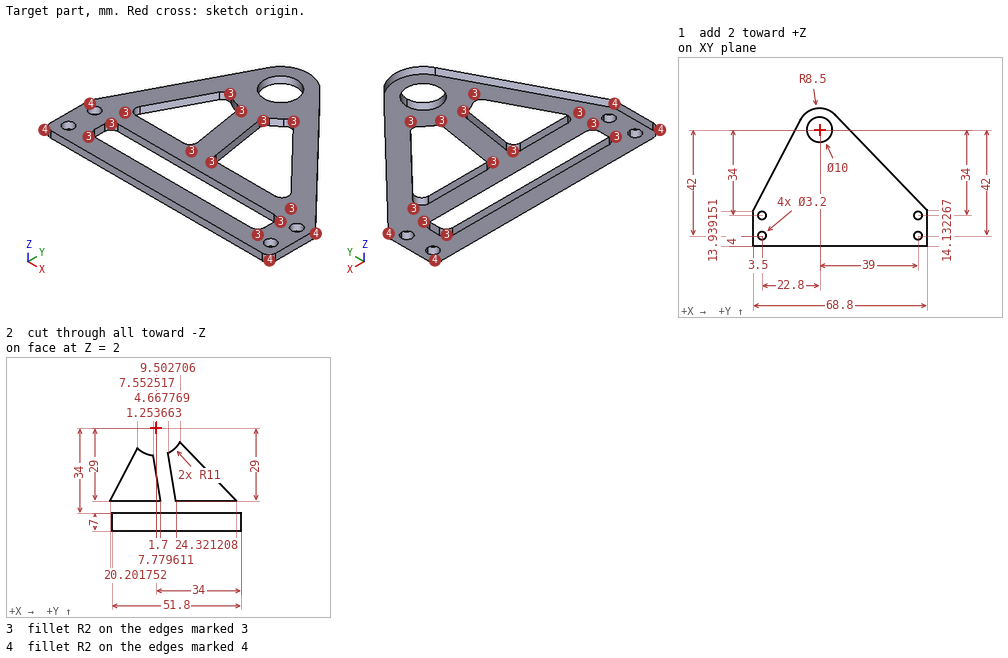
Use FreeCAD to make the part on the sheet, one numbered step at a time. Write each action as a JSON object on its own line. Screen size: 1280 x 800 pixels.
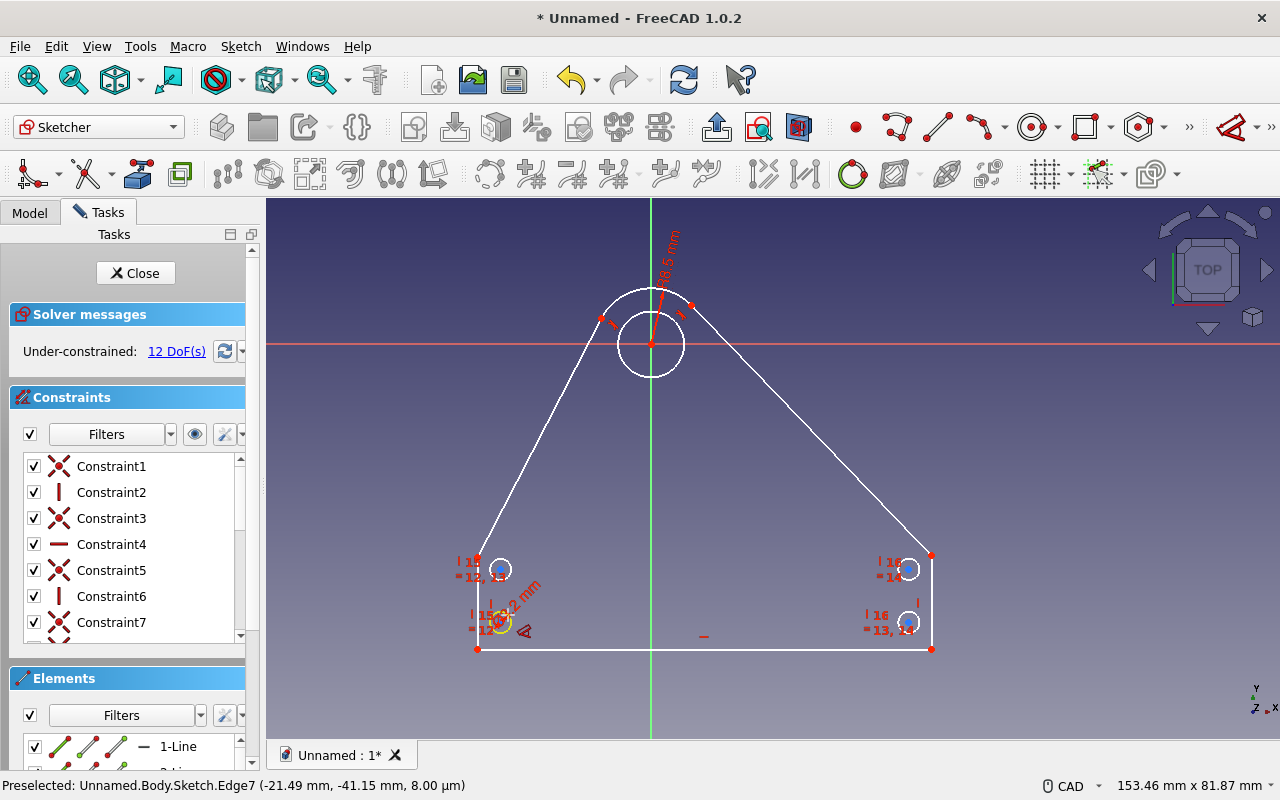
{"action": "left_click", "coordinate": [674, 321]}
{"action": "left_click", "coordinate": [698, 390]}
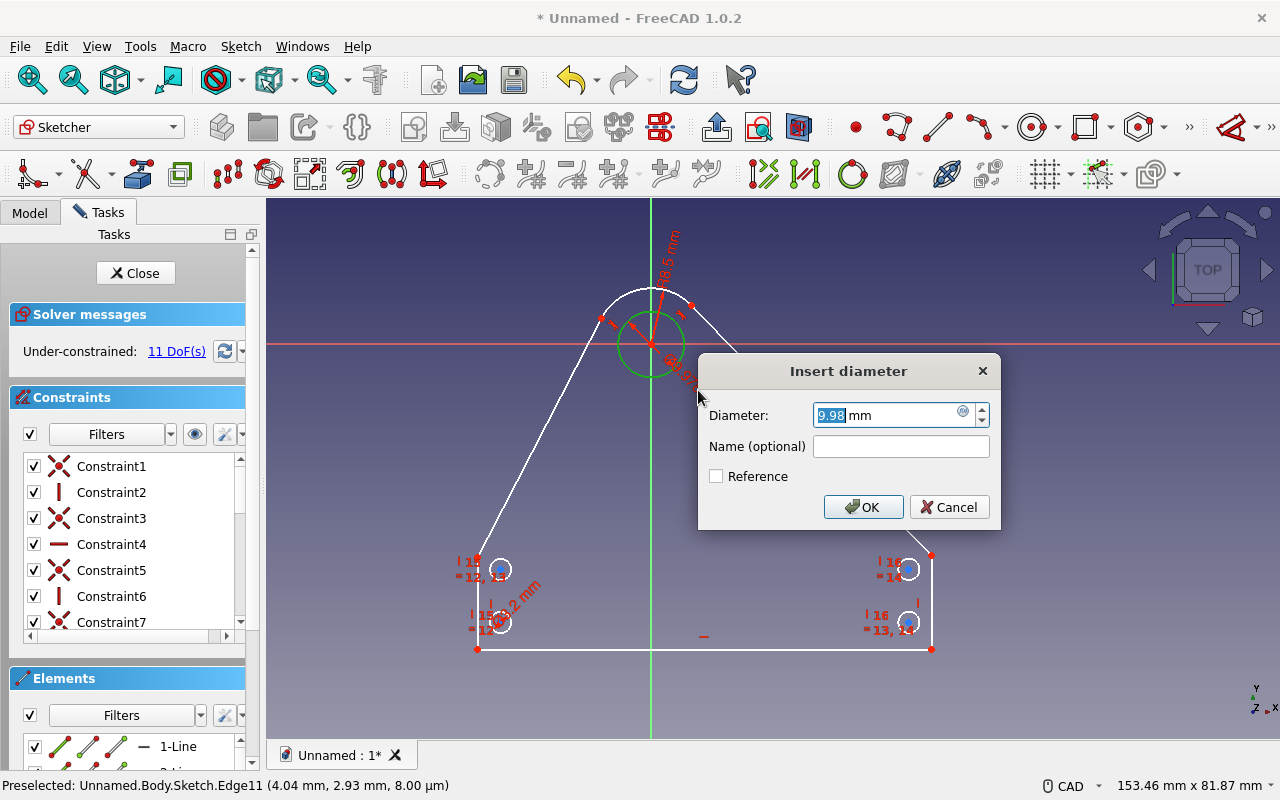
{"action": "type", "text": "10"}
{"action": "key", "text": "Return"}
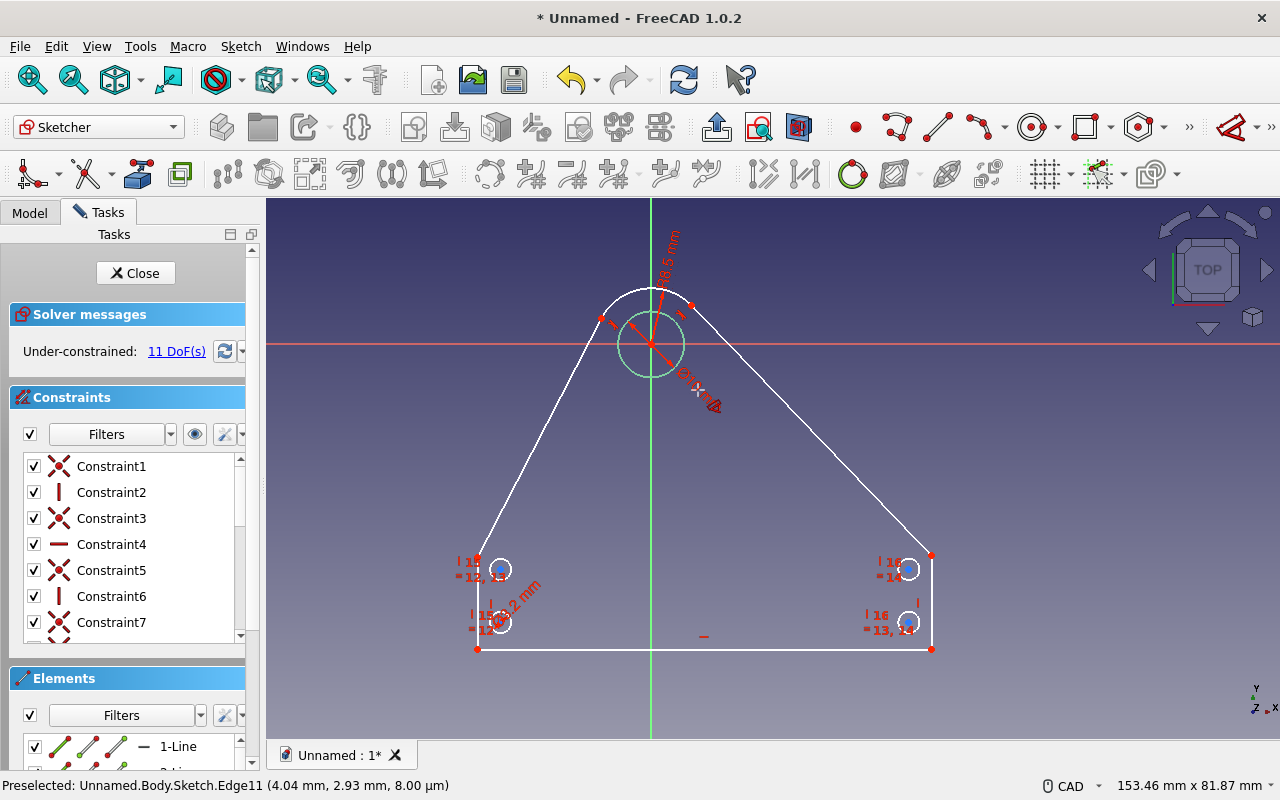
{"action": "left_click", "coordinate": [501, 623]}
{"action": "left_click", "coordinate": [467, 484]}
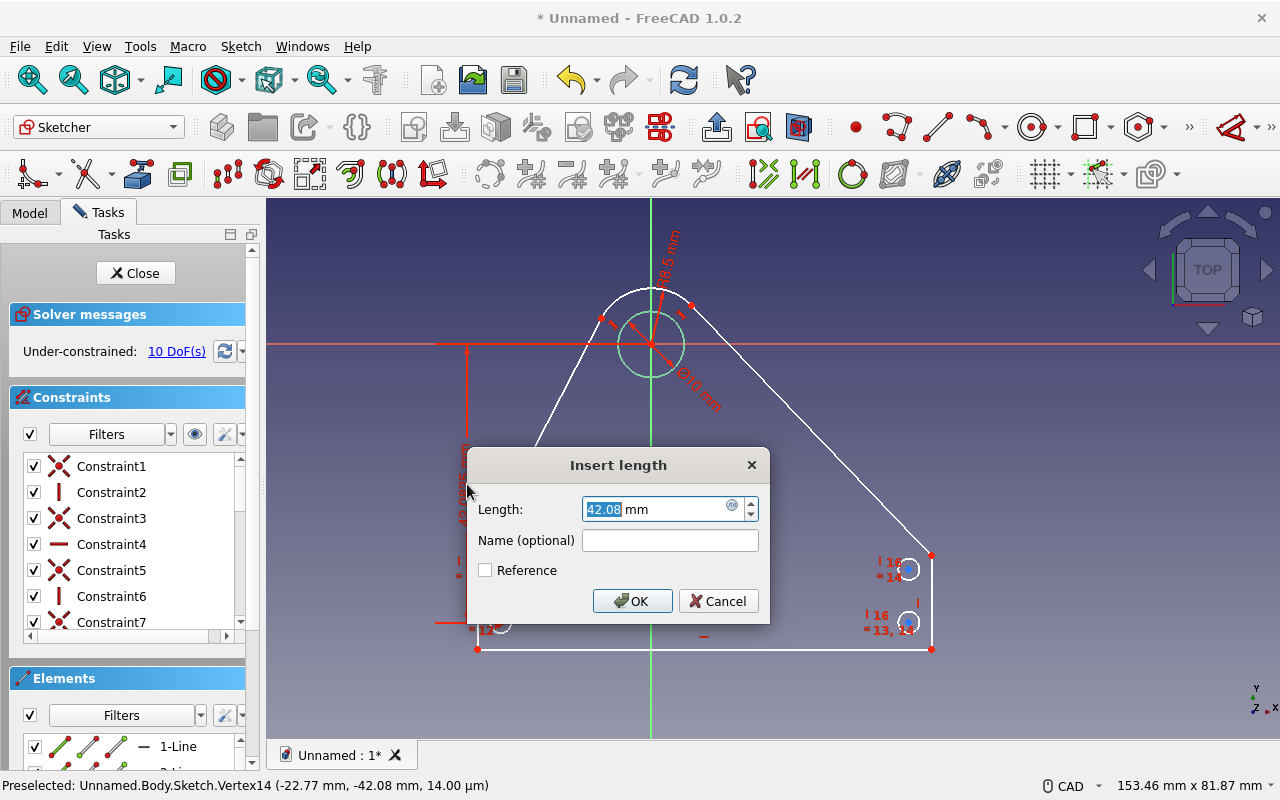
{"action": "type", "text": "42"}
{"action": "key", "text": "Return"}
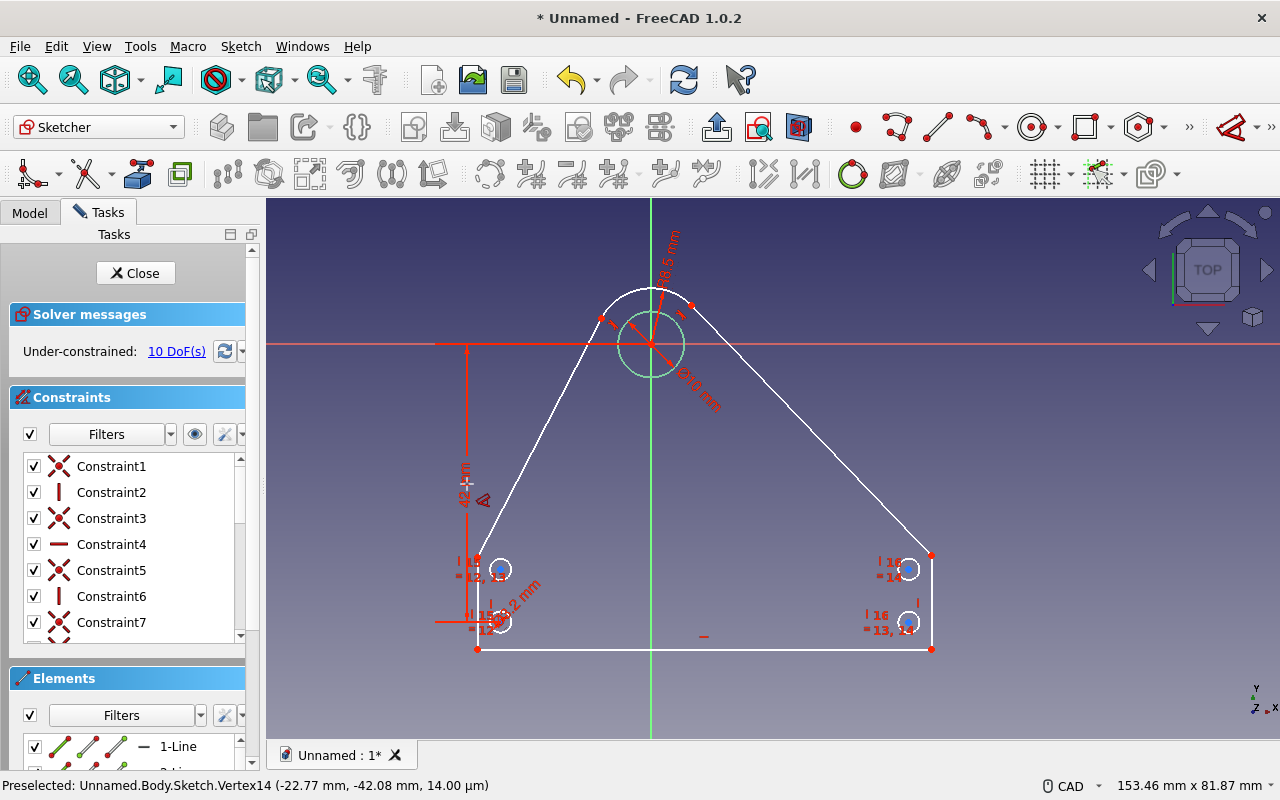
{"action": "left_click", "coordinate": [501, 570]}
{"action": "left_click", "coordinate": [467, 457]}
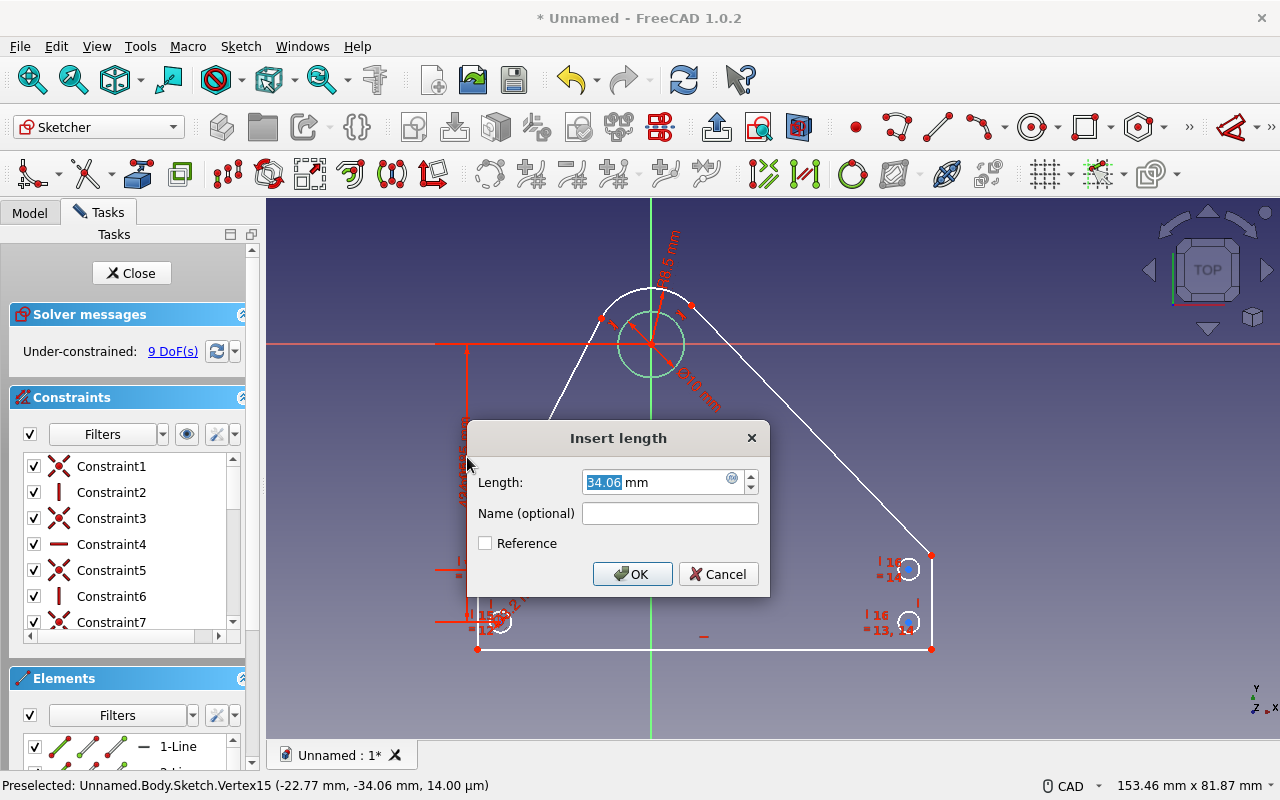
{"action": "type", "text": "34"}
{"action": "key", "text": "Return"}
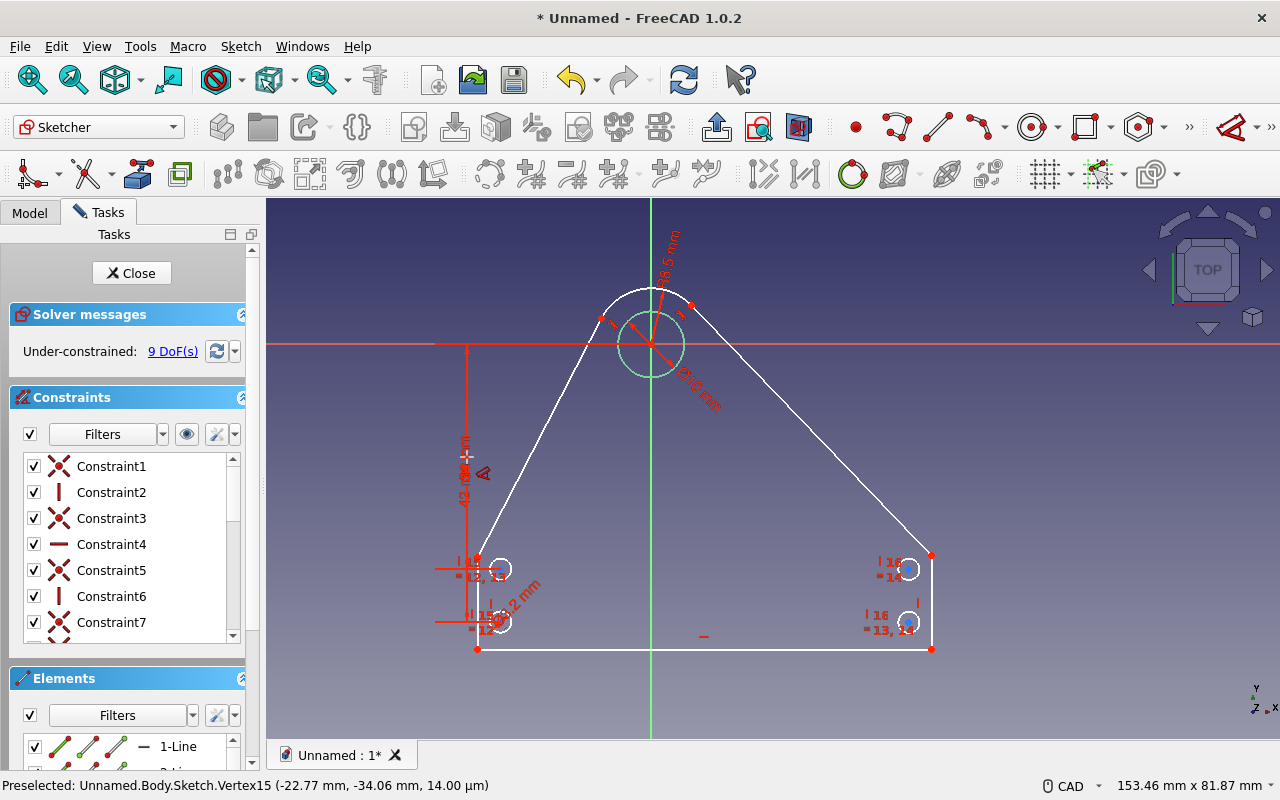
{"action": "left_click", "coordinate": [909, 622]}
{"action": "left_click", "coordinate": [780, 310]}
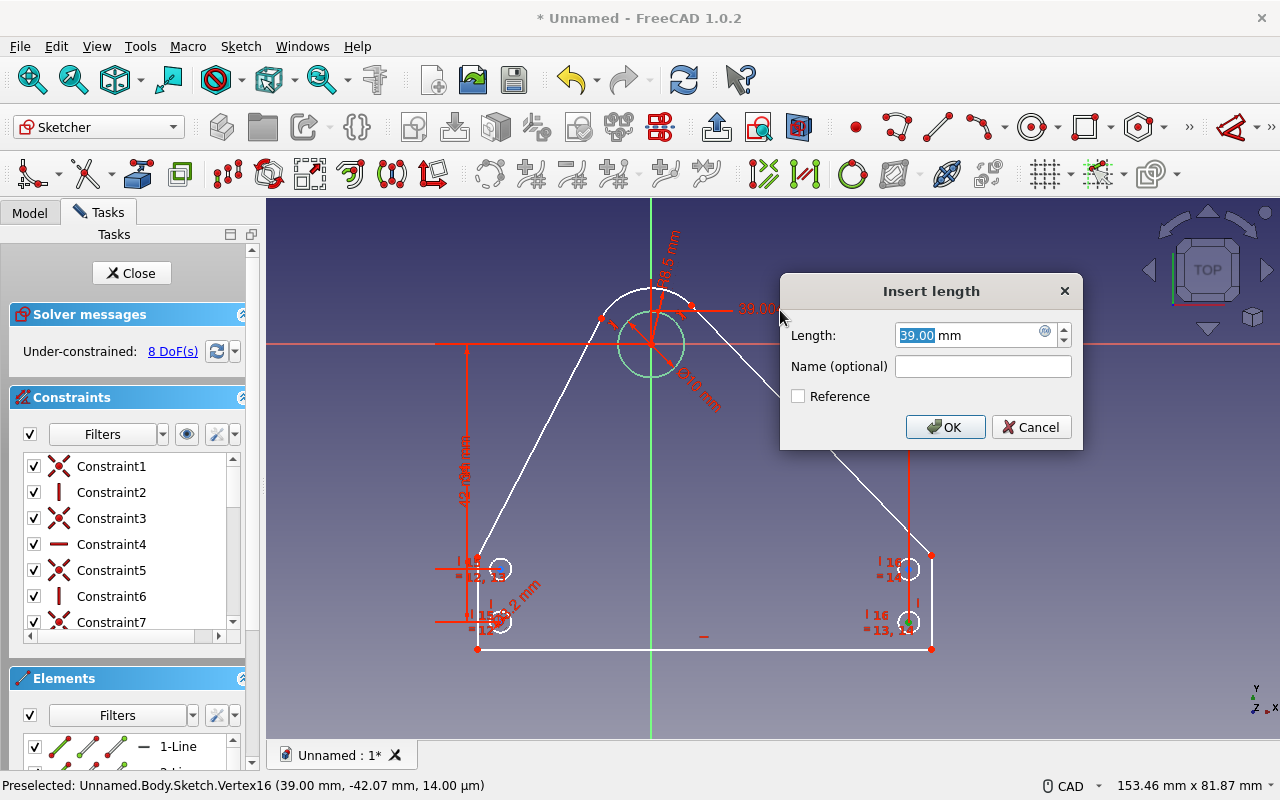
{"action": "type", "text": "39"}
{"action": "key", "text": "Return"}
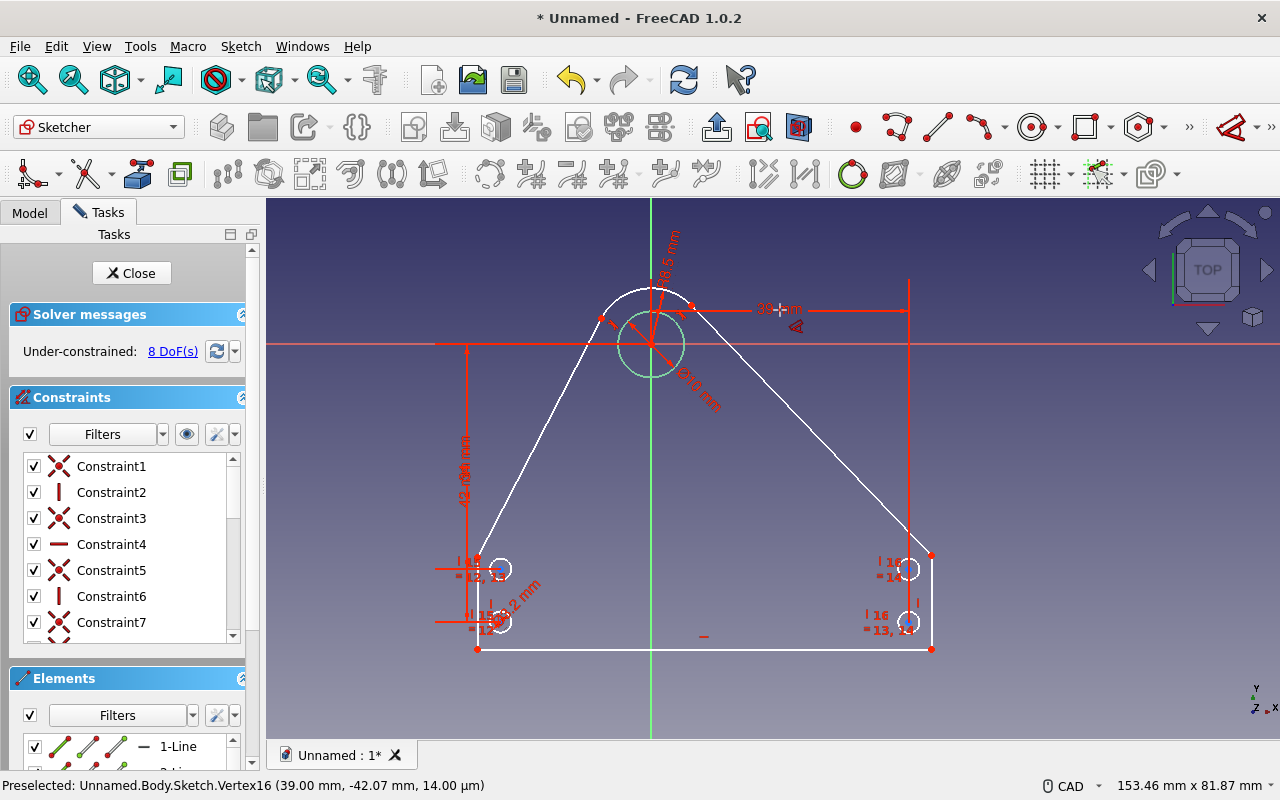
{"action": "left_click", "coordinate": [909, 622]}
{"action": "left_click", "coordinate": [943, 483]}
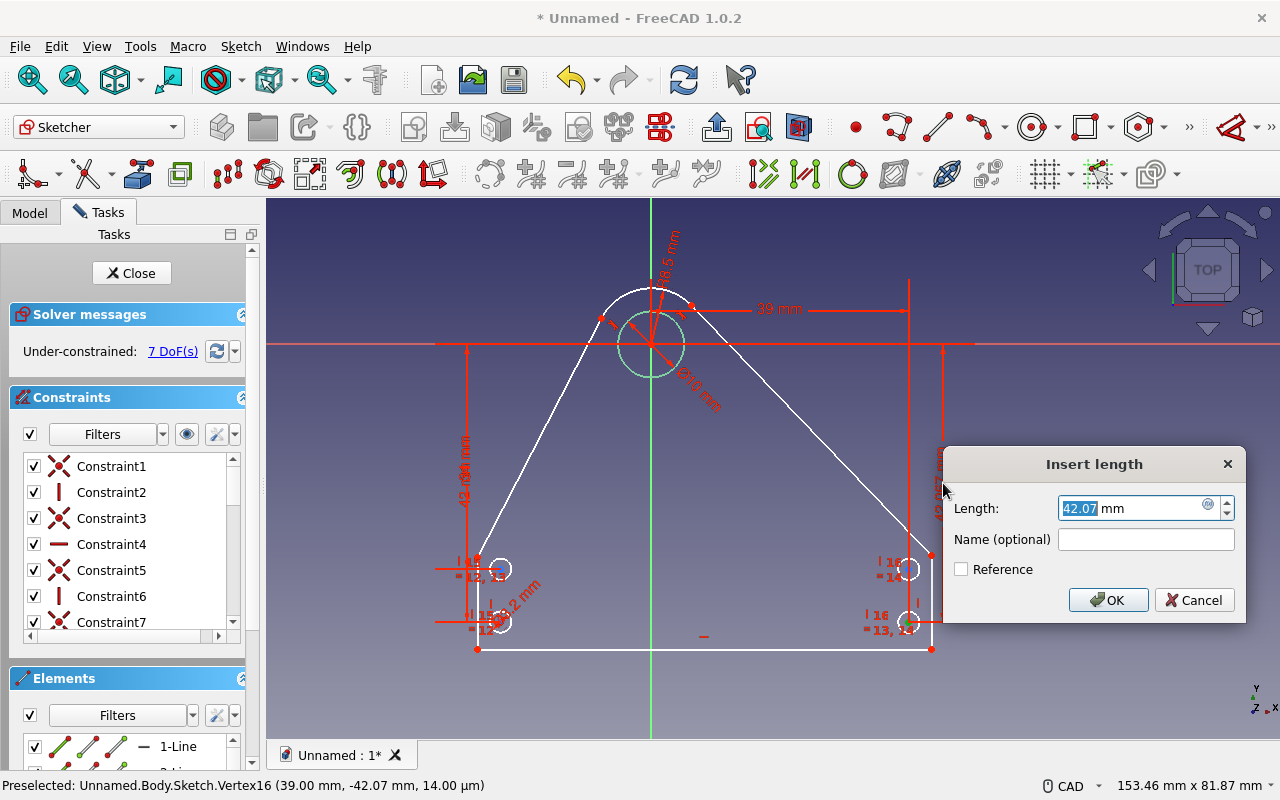
{"action": "type", "text": "42"}
{"action": "key", "text": "Return"}